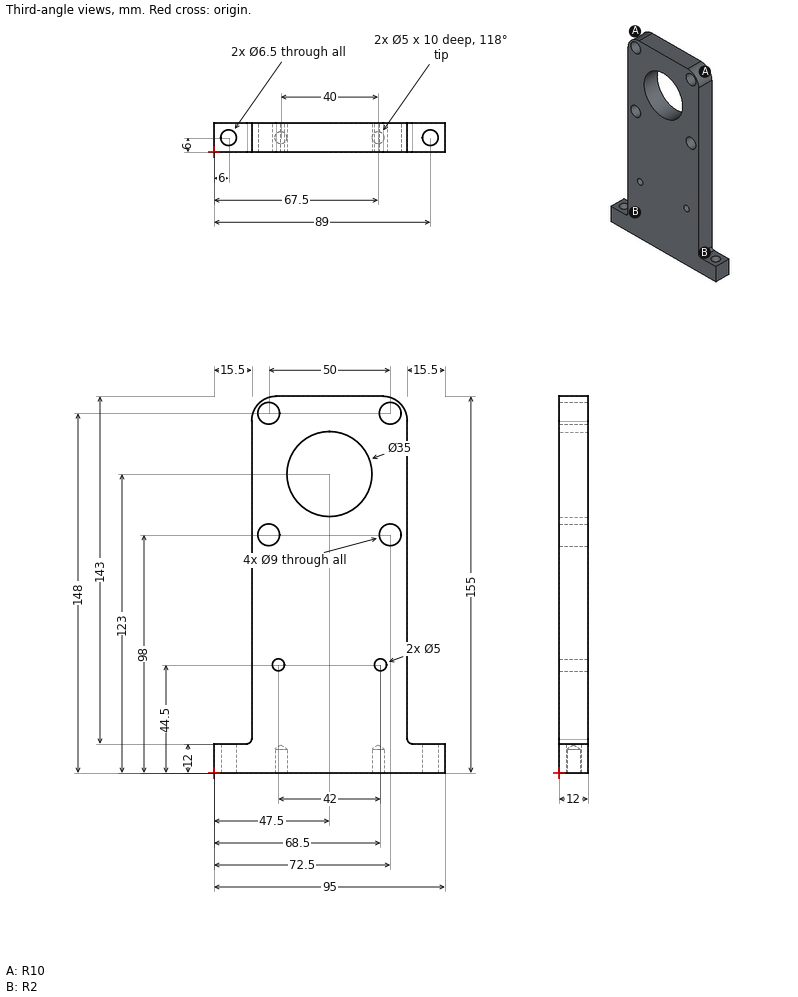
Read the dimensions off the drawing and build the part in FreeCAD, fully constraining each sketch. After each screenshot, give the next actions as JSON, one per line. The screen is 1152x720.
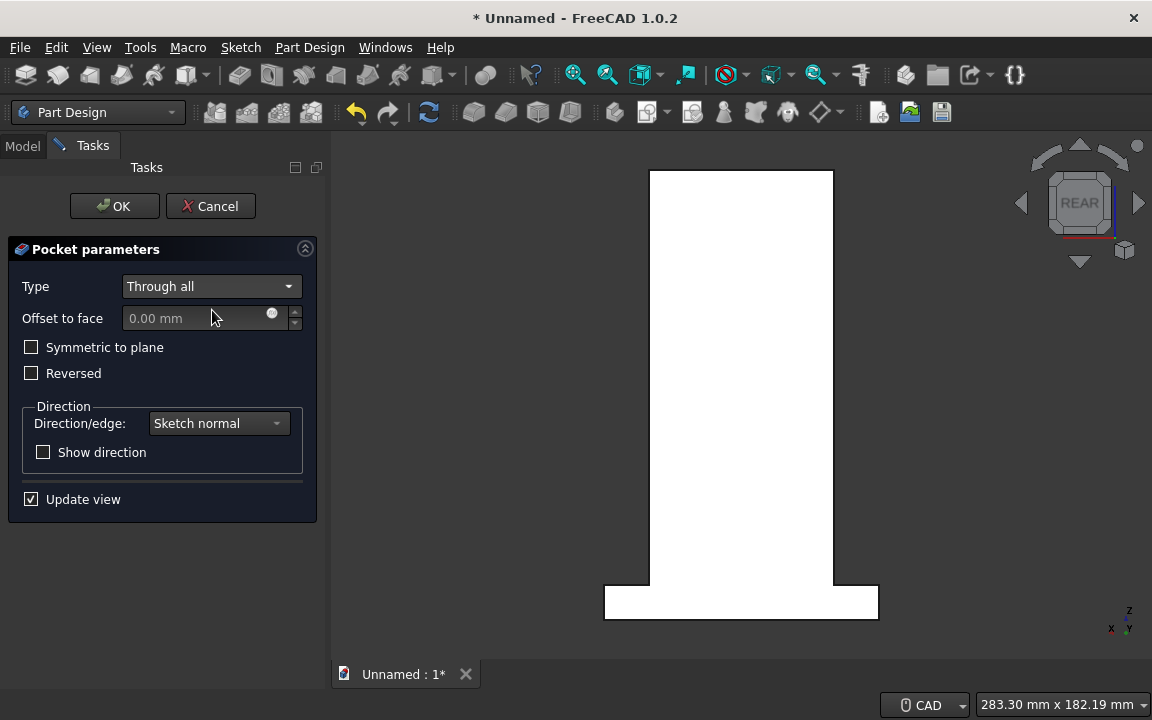
{"action": "left_click", "coordinate": [115, 206]}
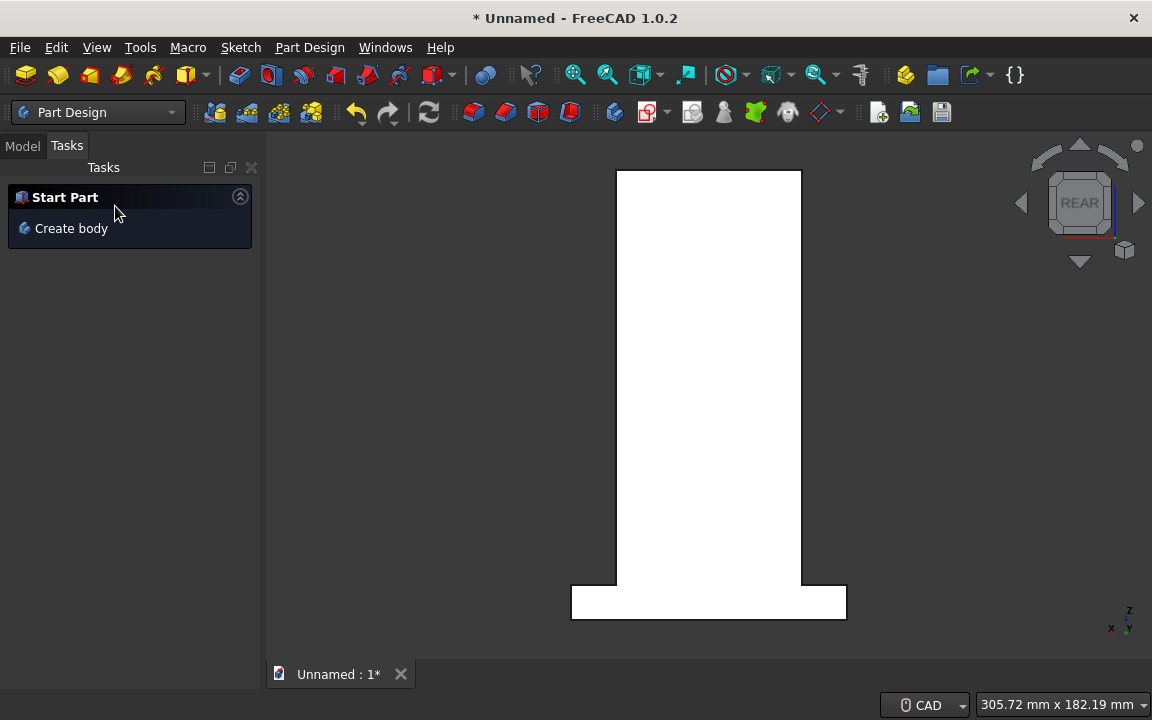
{"action": "key", "text": "0"}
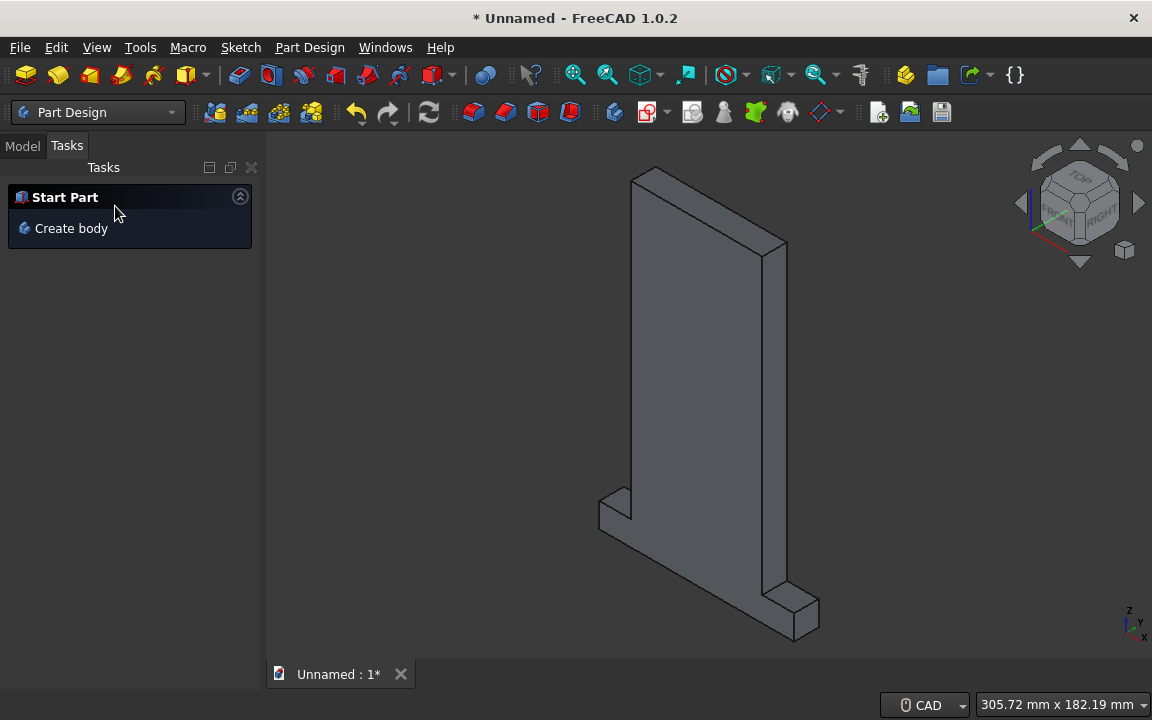
{"action": "left_click", "coordinate": [623, 499]}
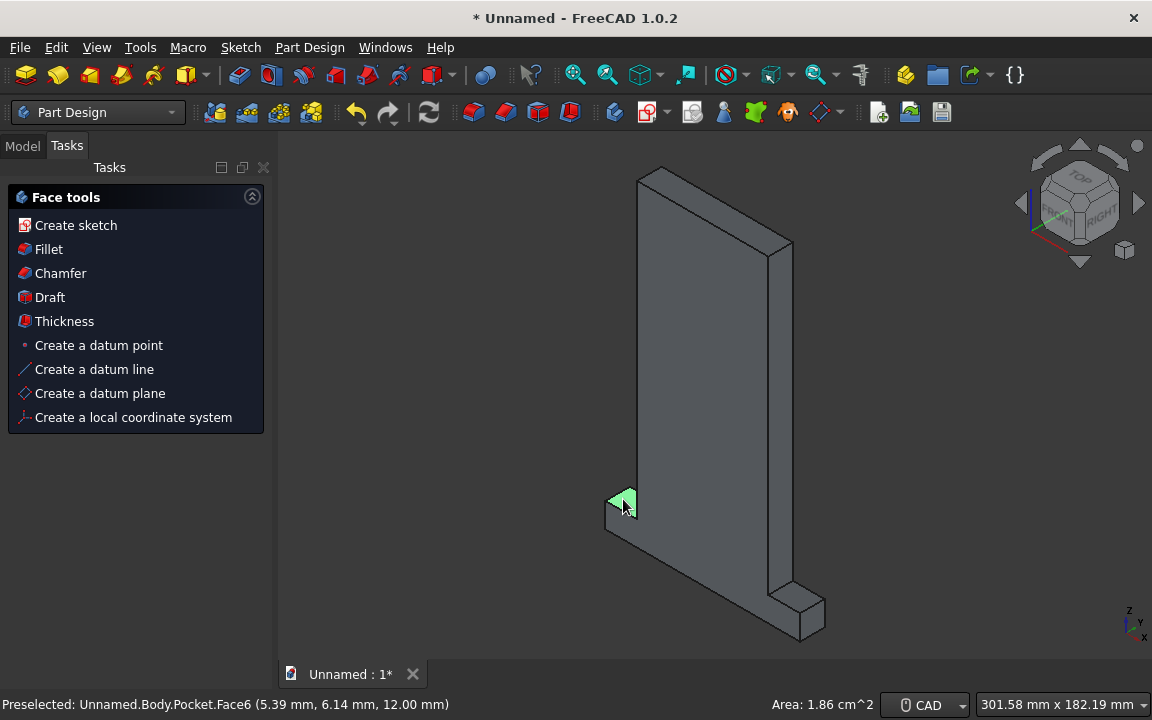
{"action": "left_click", "coordinate": [648, 112]}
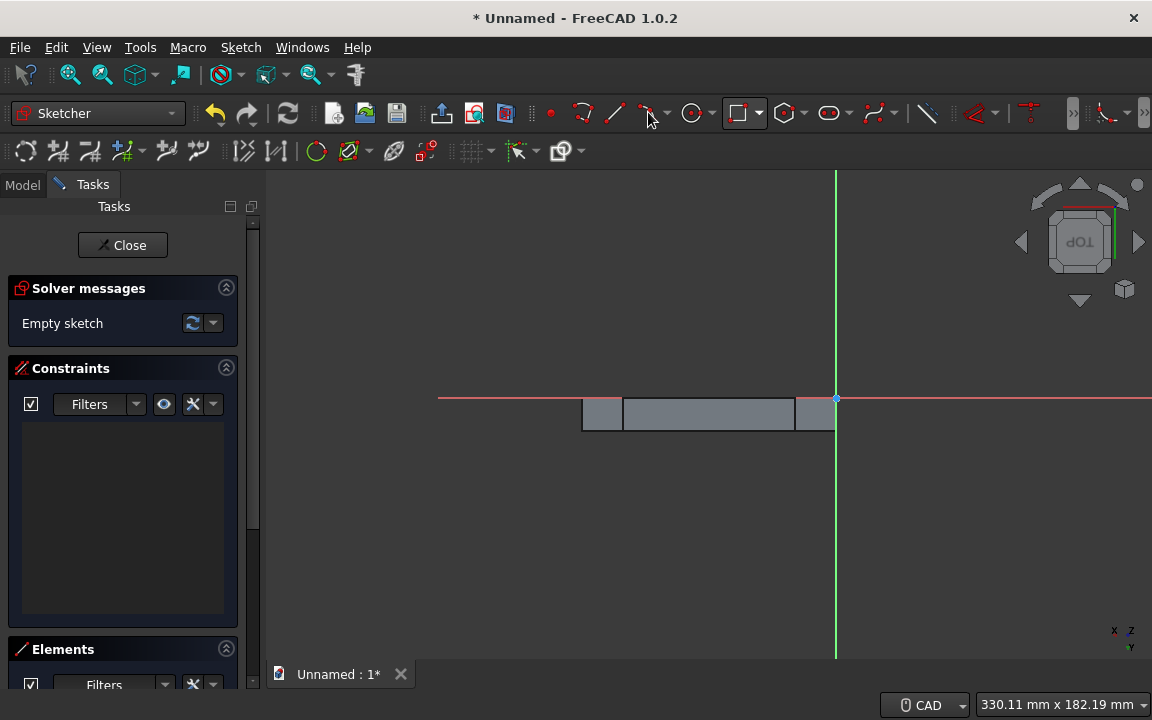
{"action": "scroll", "coordinate": [801, 406], "scroll_direction": "up", "scroll_amount": 3}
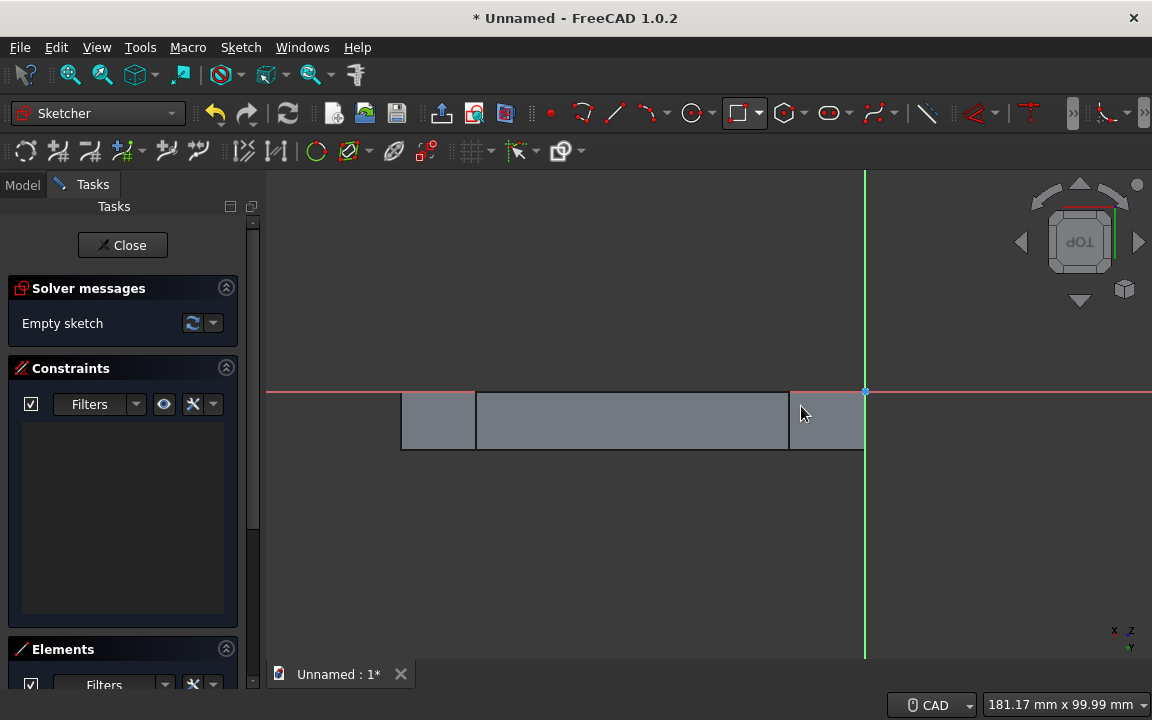
{"action": "key", "text": "g c"}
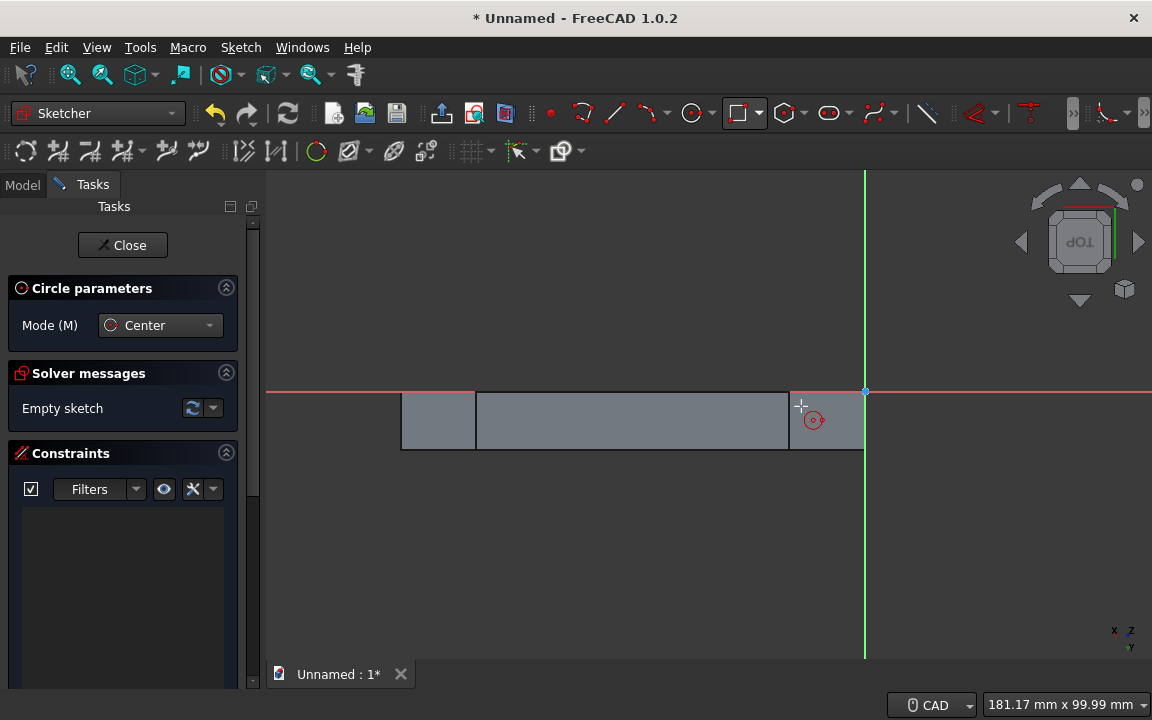
{"action": "scroll", "coordinate": [836, 421], "scroll_direction": "up", "scroll_amount": 2}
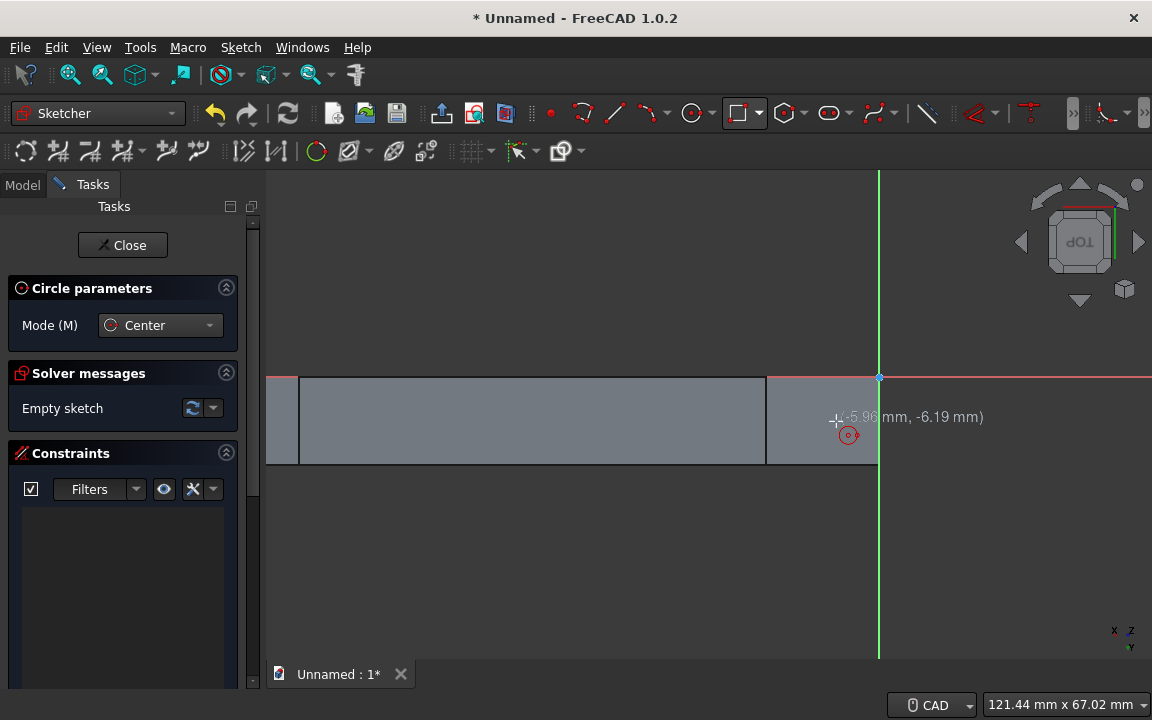
{"action": "left_click", "coordinate": [835, 421]}
{"action": "left_click", "coordinate": [852, 404]}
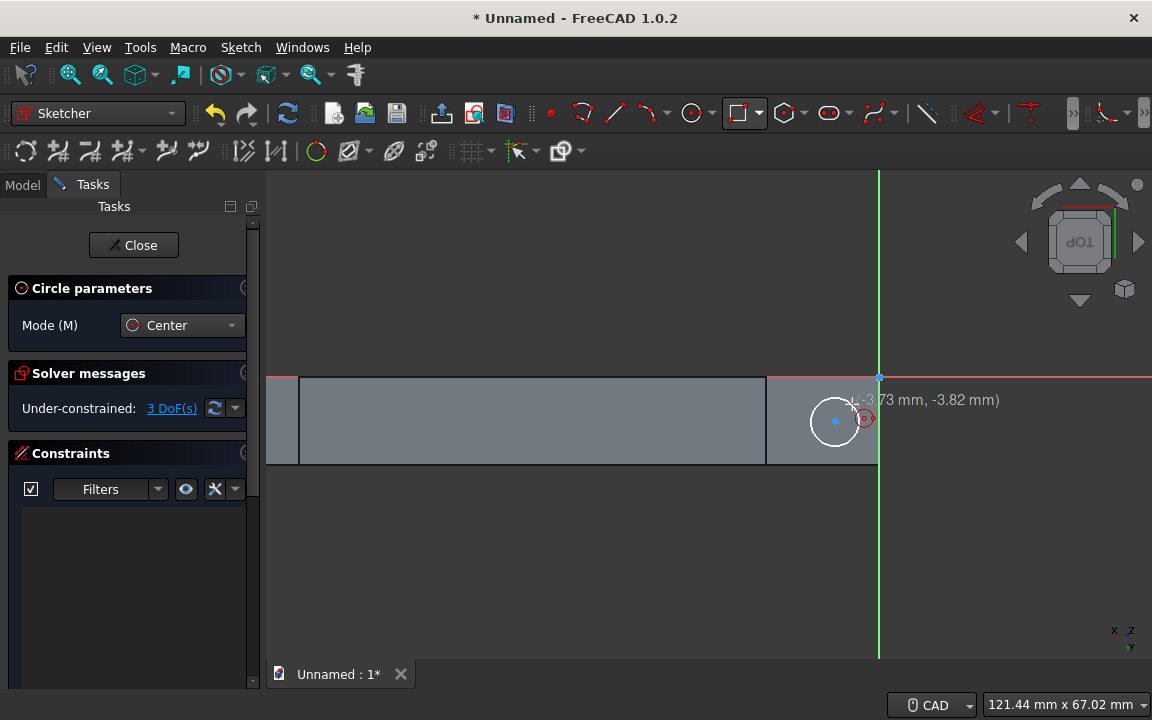
{"action": "scroll", "coordinate": [839, 422], "scroll_direction": "down", "scroll_amount": 2}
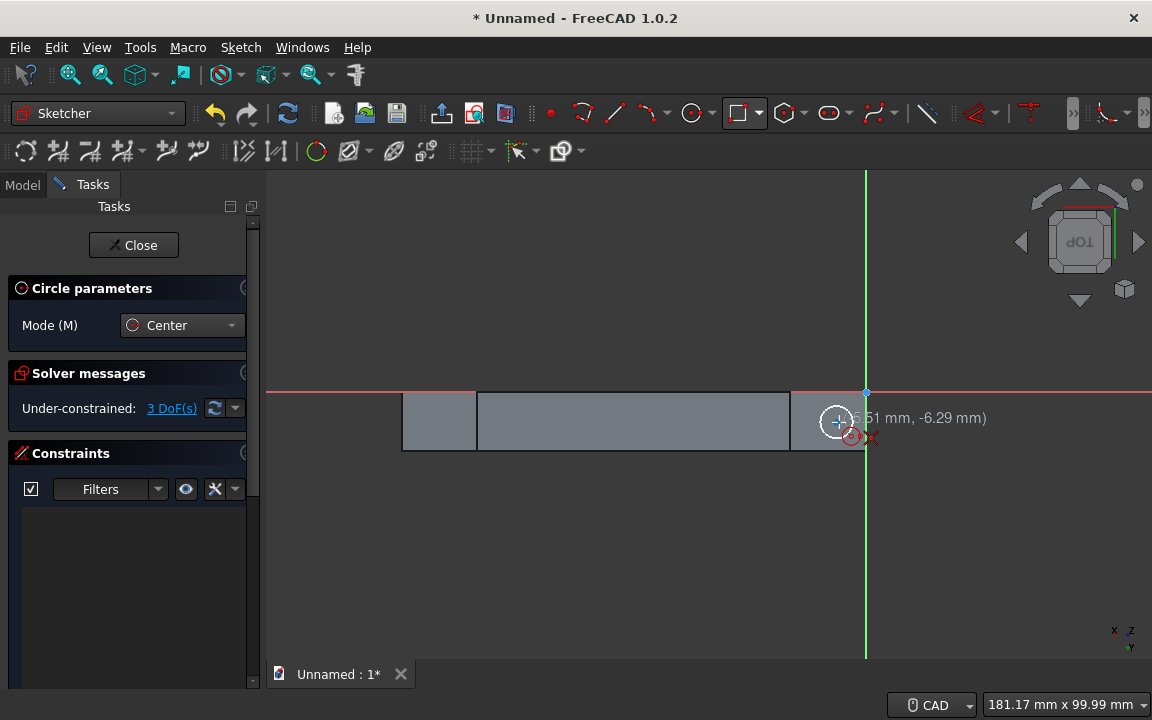
{"action": "scroll", "coordinate": [431, 421], "scroll_direction": "up", "scroll_amount": 2}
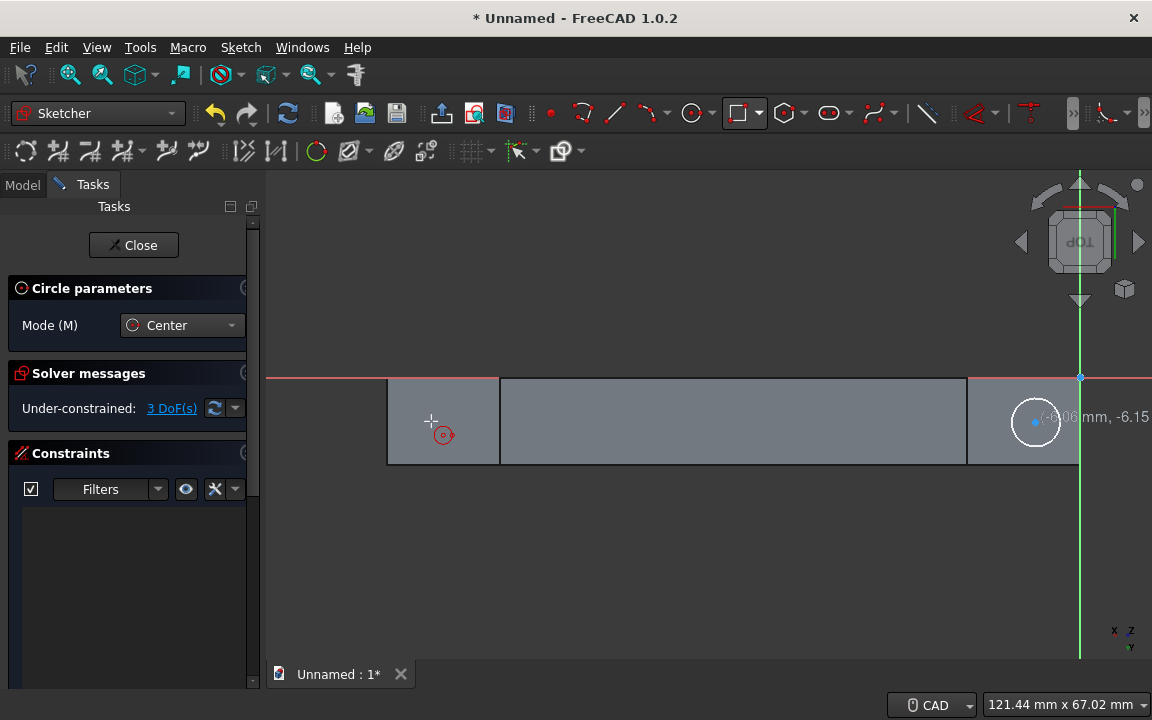
{"action": "left_click", "coordinate": [431, 421]}
{"action": "left_click", "coordinate": [448, 405]}
{"action": "key", "text": "Escape"}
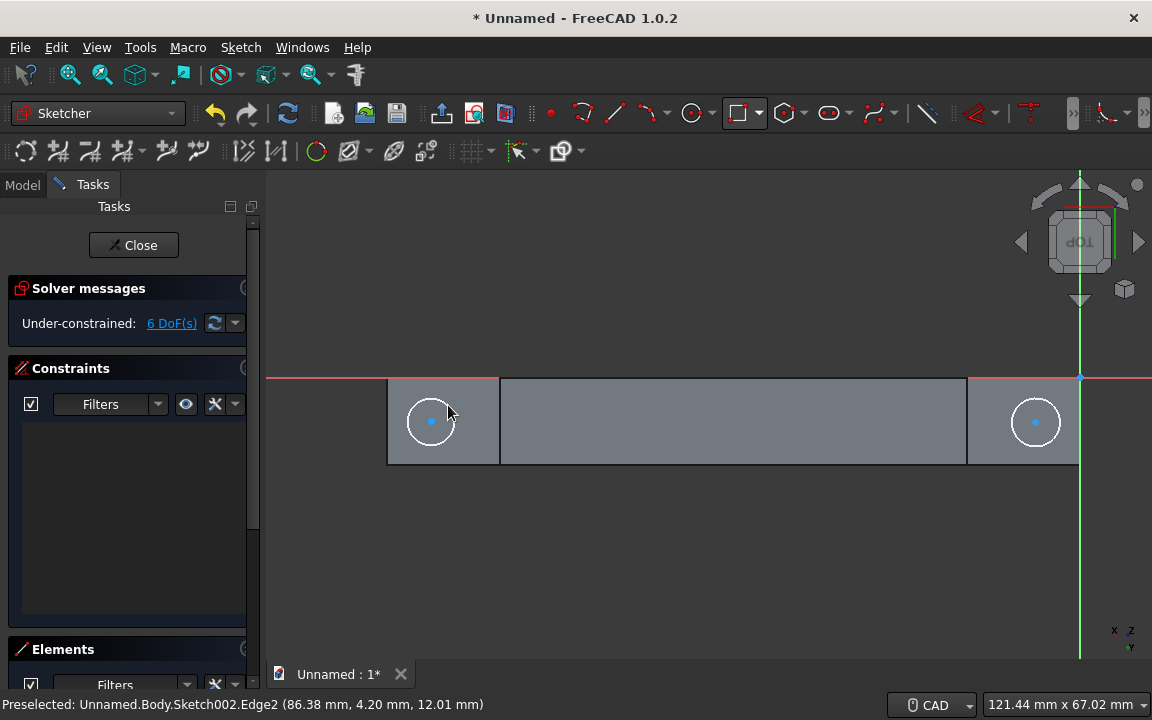
{"action": "scroll", "coordinate": [431, 421], "scroll_direction": "down", "scroll_amount": 2}